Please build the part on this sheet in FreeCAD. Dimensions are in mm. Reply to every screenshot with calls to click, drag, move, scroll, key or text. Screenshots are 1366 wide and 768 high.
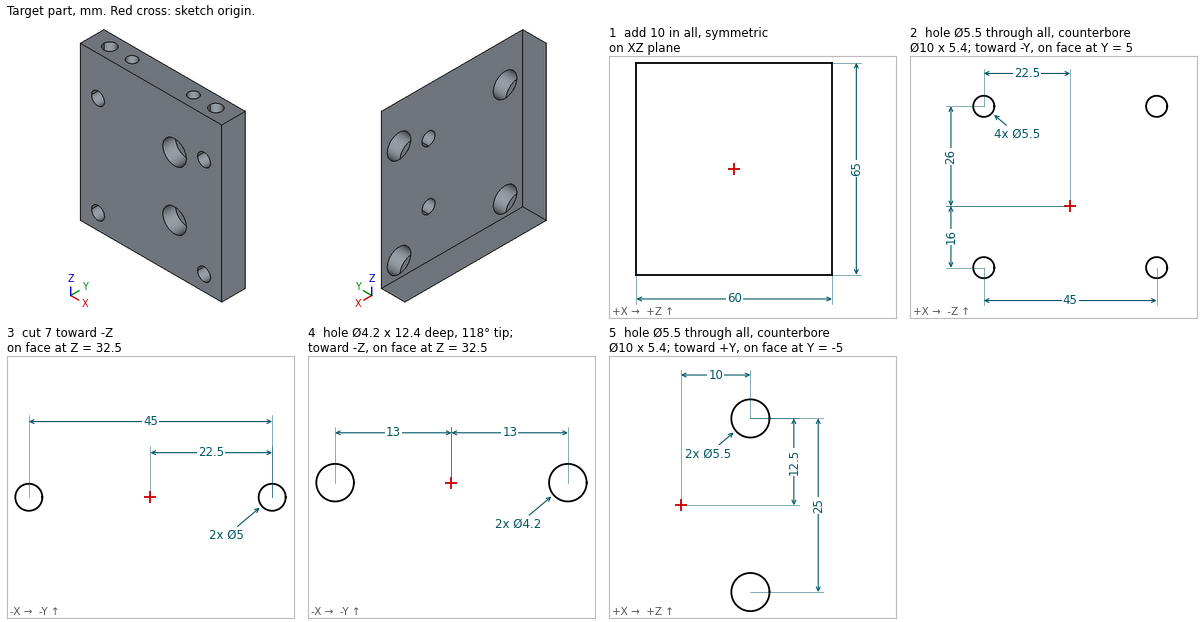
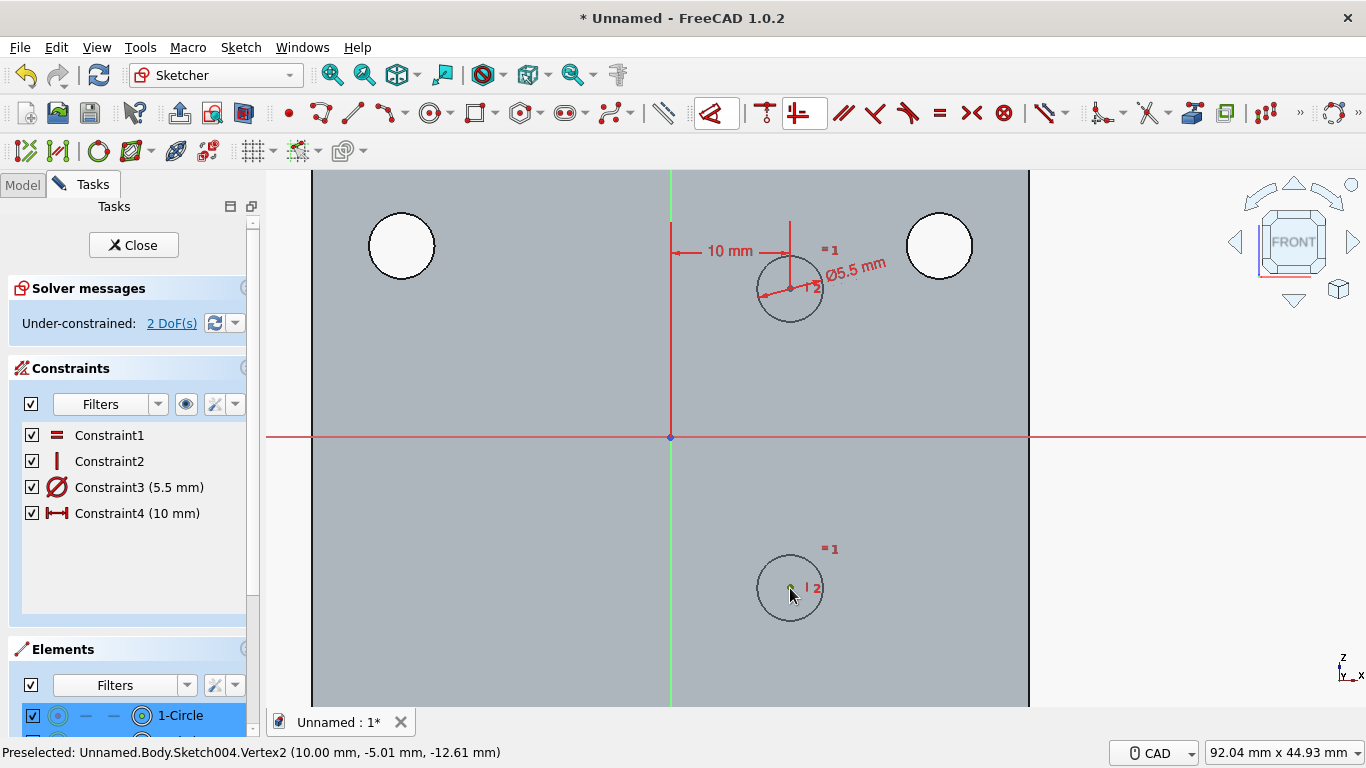
key(i)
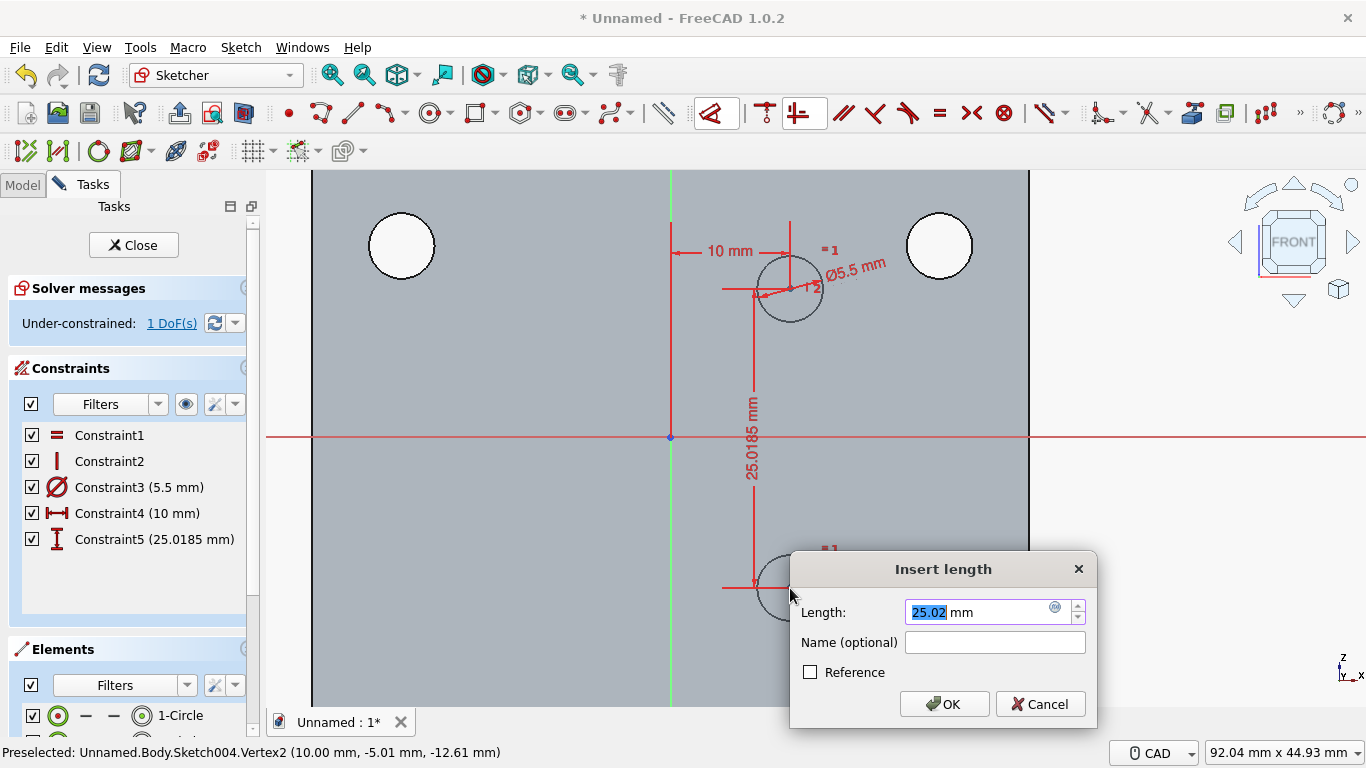
text(25)
key(Return)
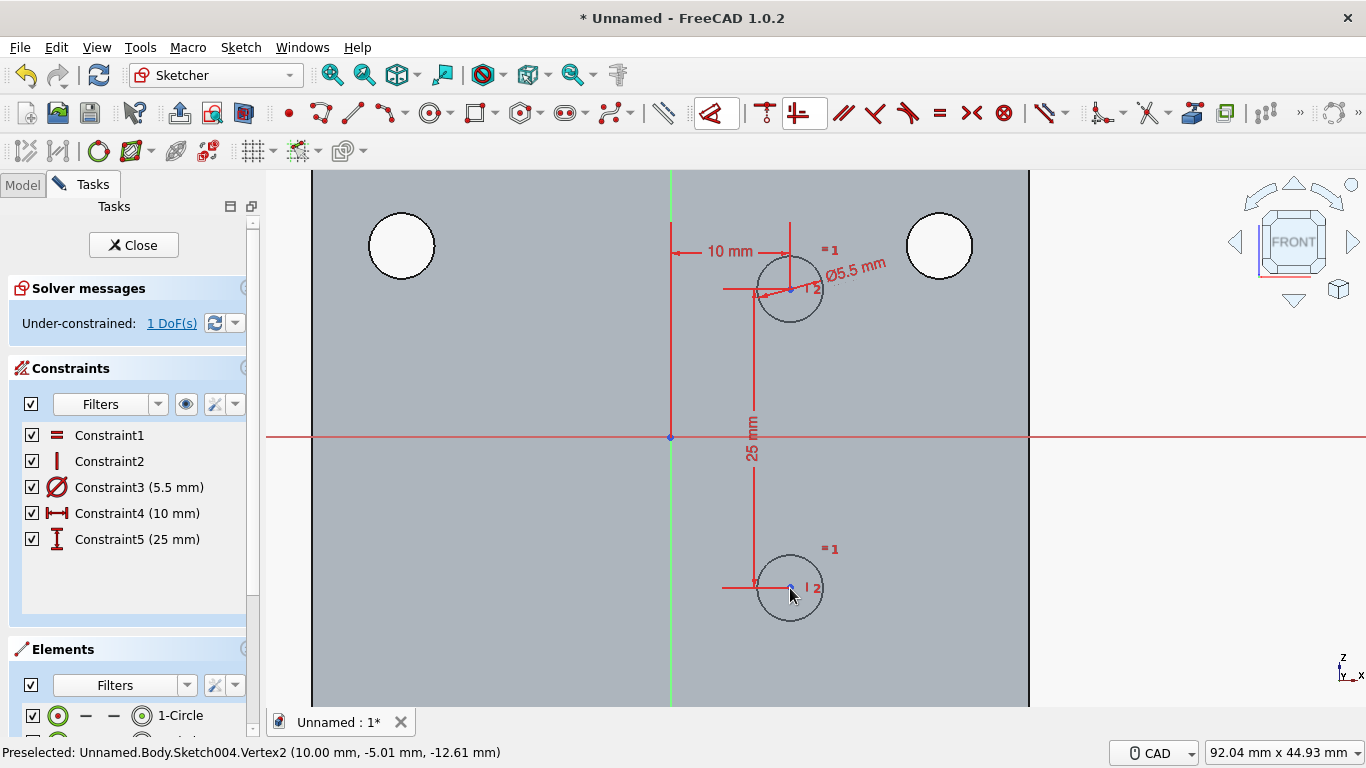
click(790, 289)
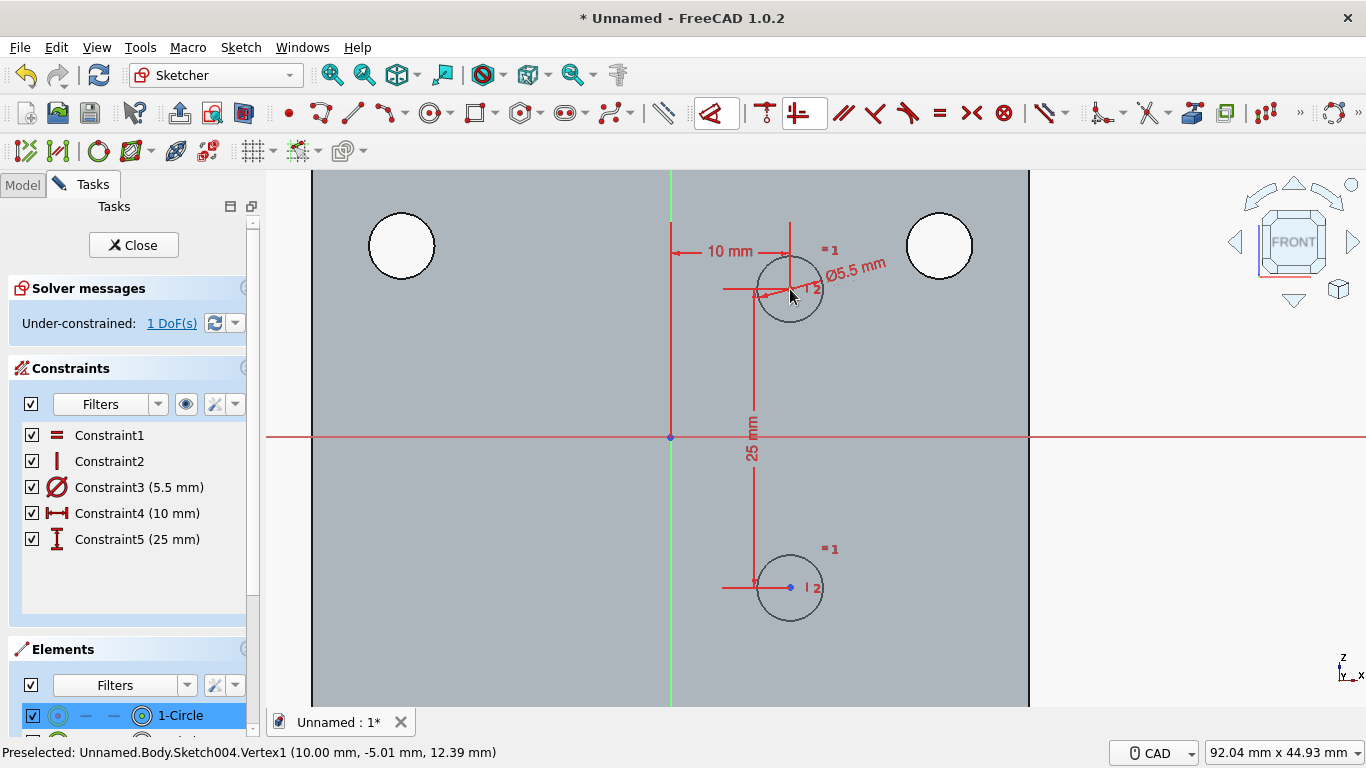
key(i)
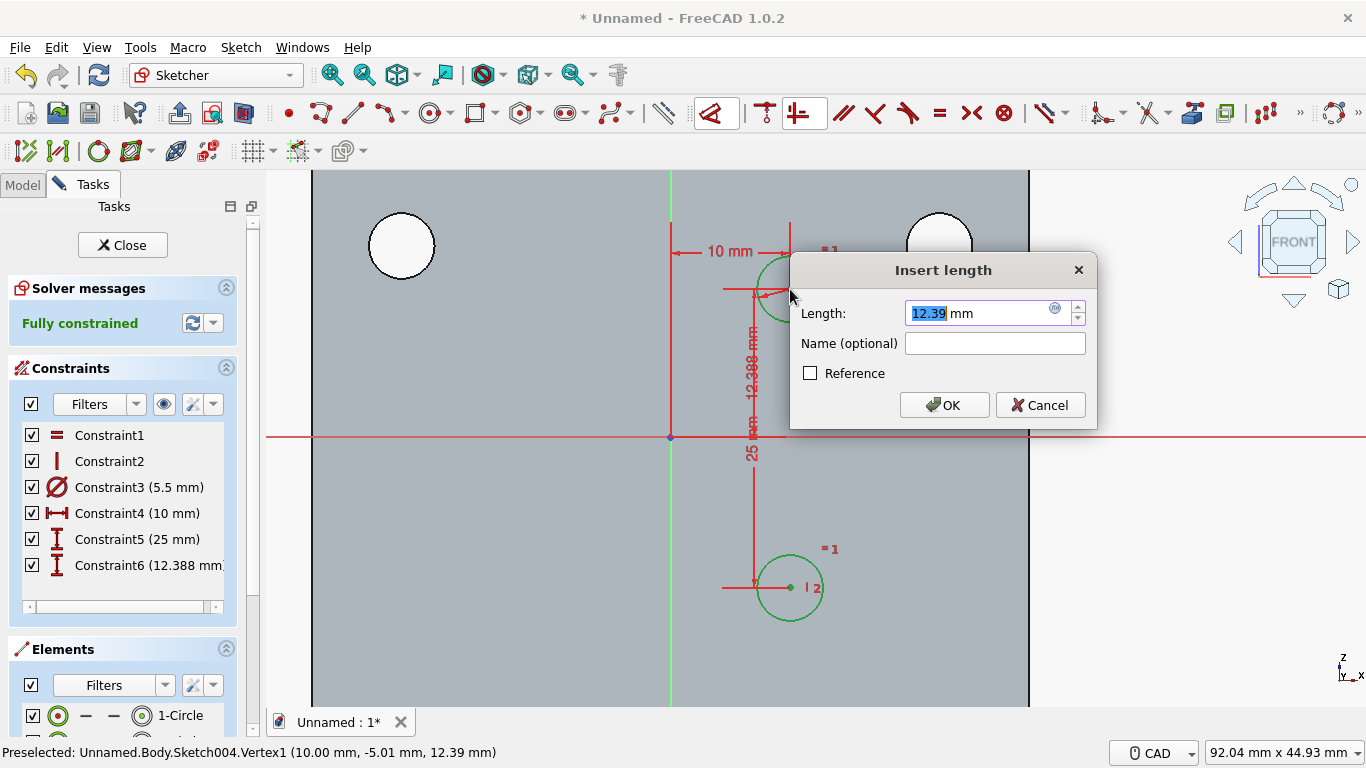
text(12.5)
key(Return)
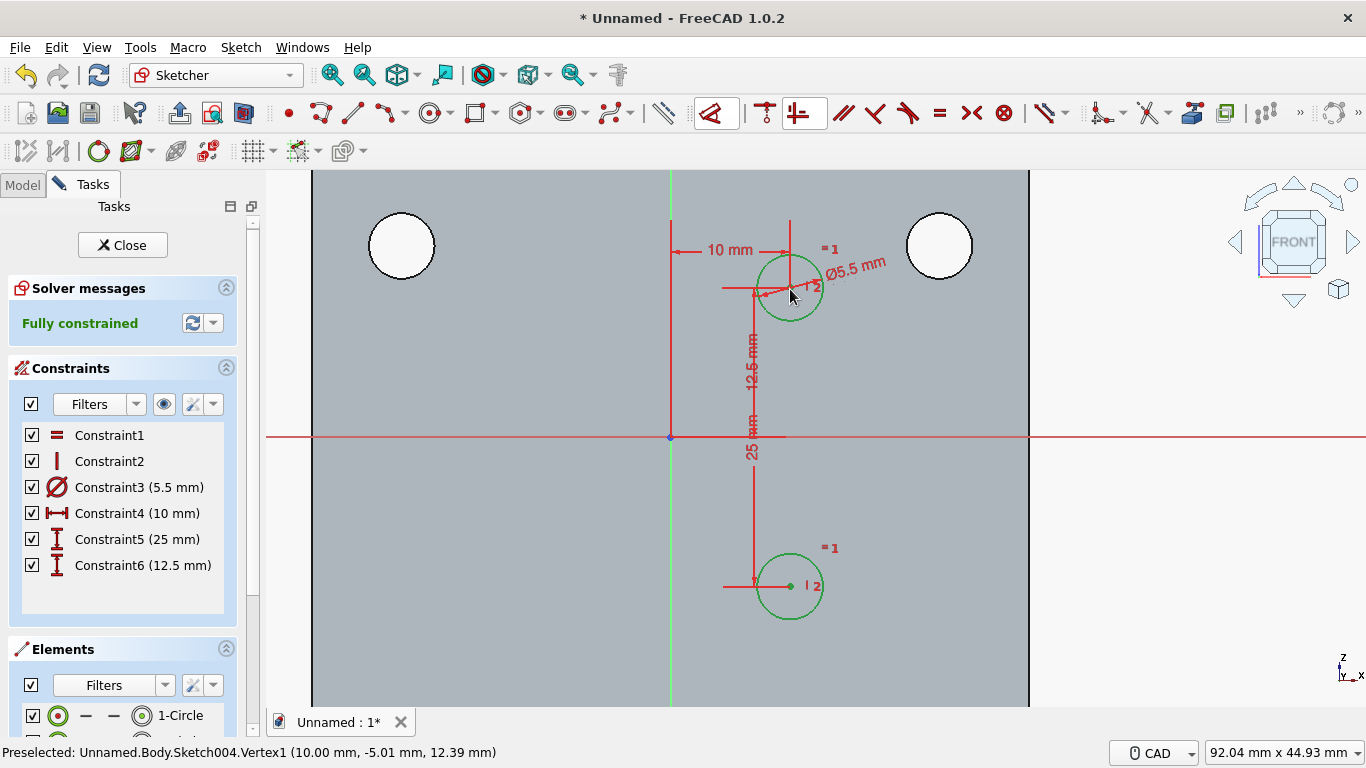
click(123, 245)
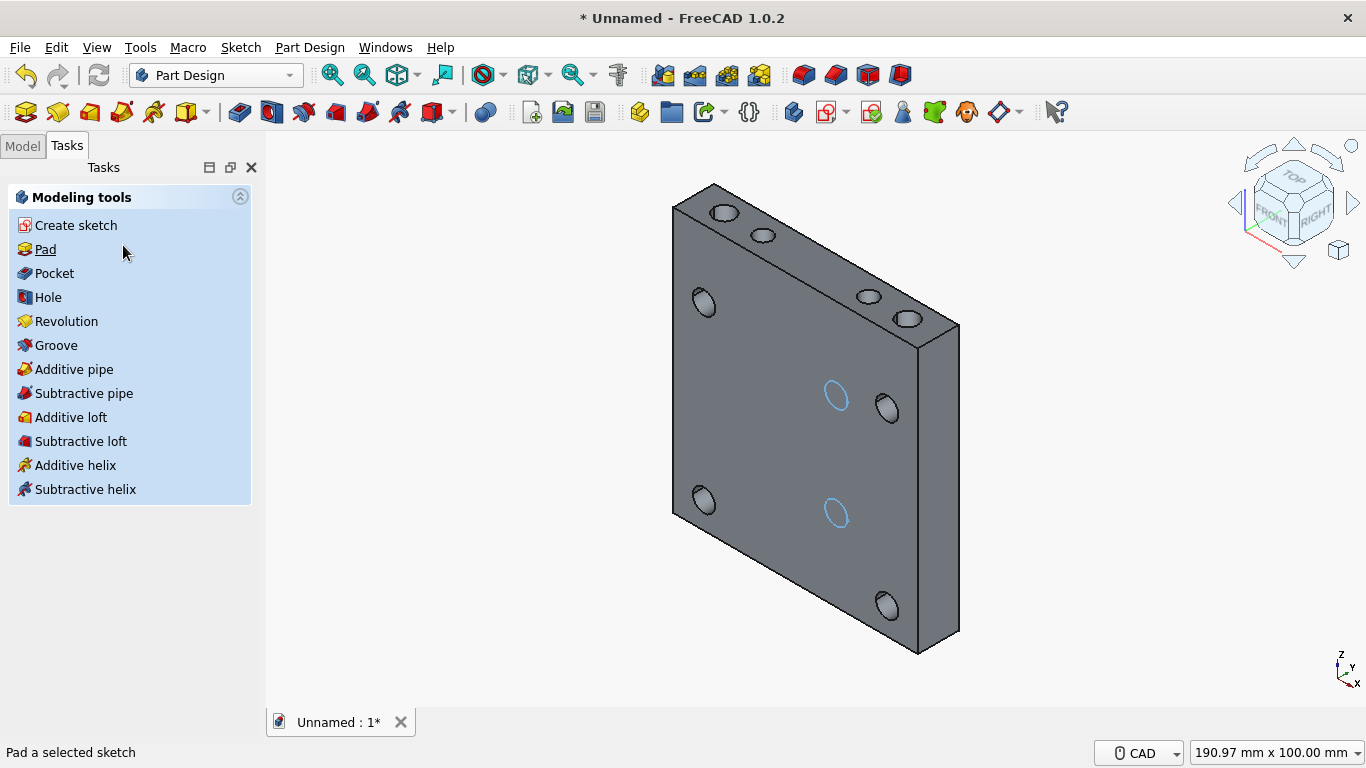
click(272, 112)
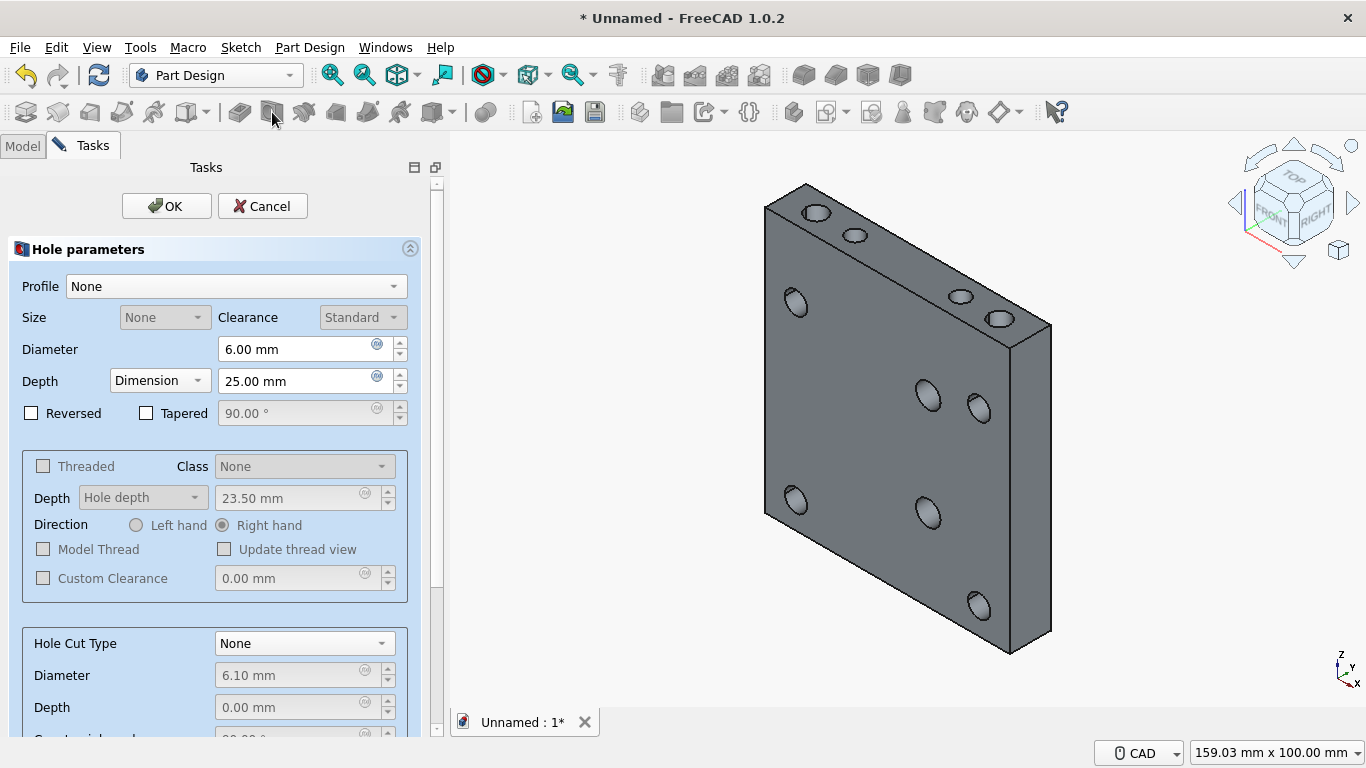
triple_click(305, 349)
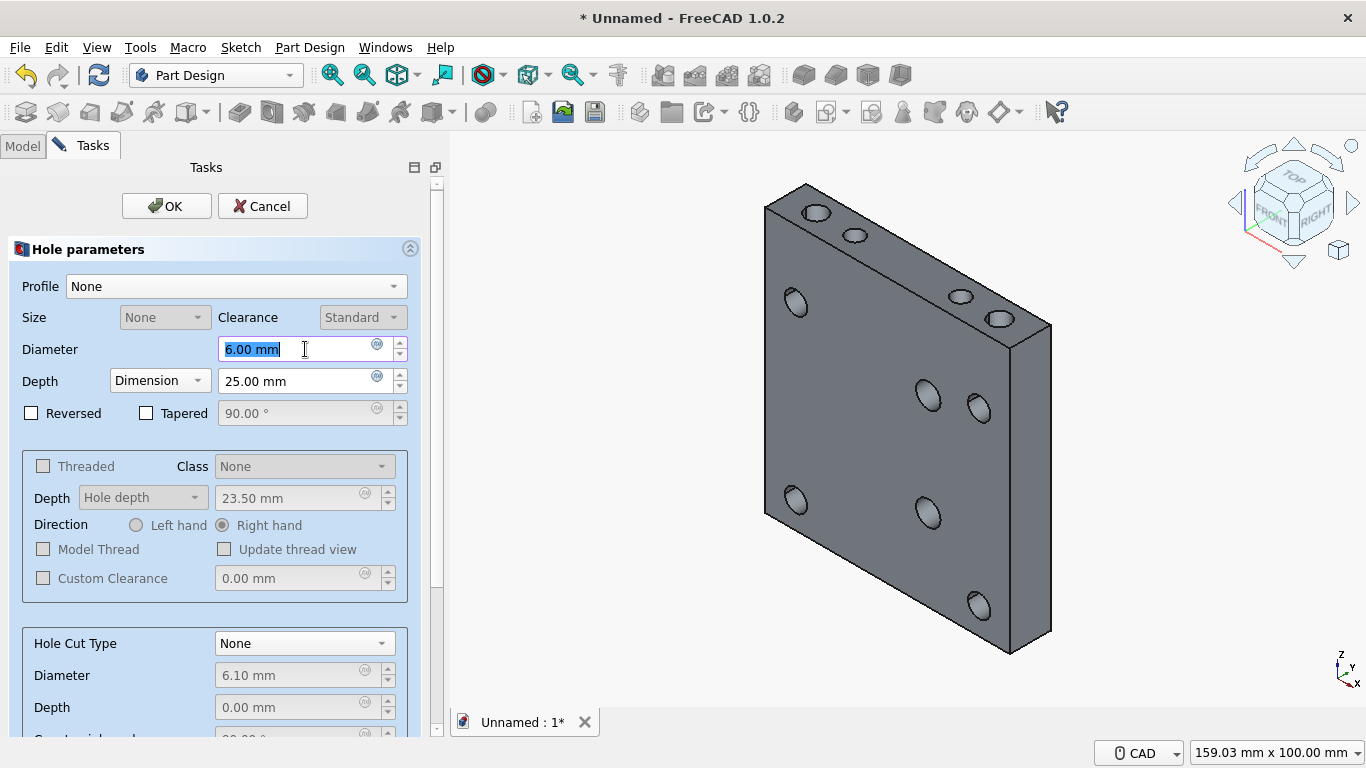
text(5.5)
key(Tab)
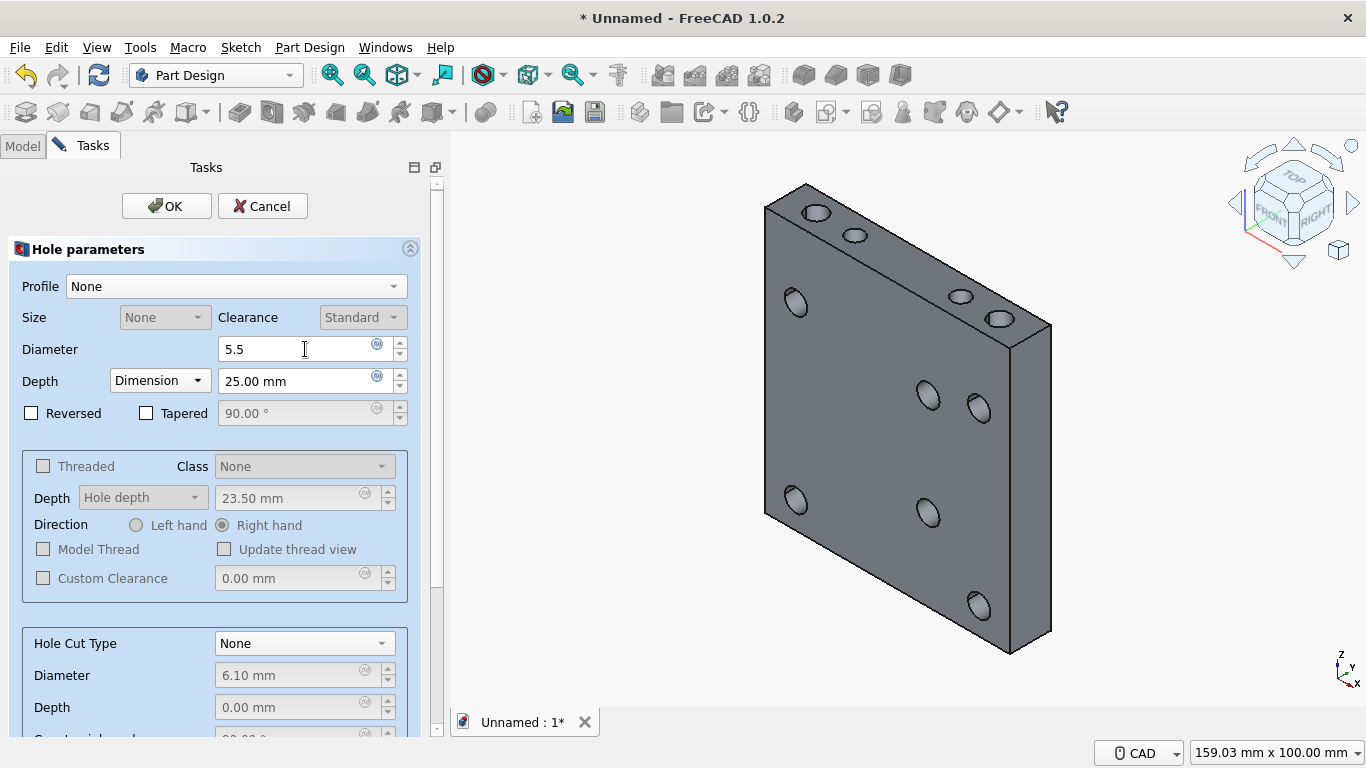
click(161, 380)